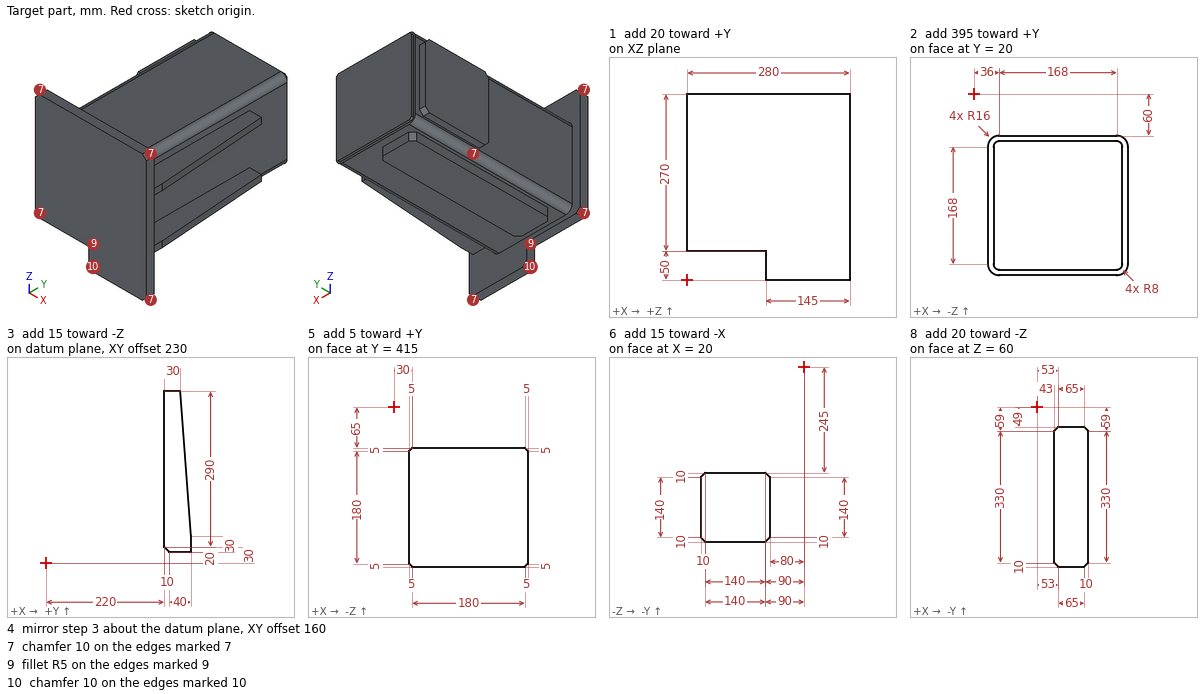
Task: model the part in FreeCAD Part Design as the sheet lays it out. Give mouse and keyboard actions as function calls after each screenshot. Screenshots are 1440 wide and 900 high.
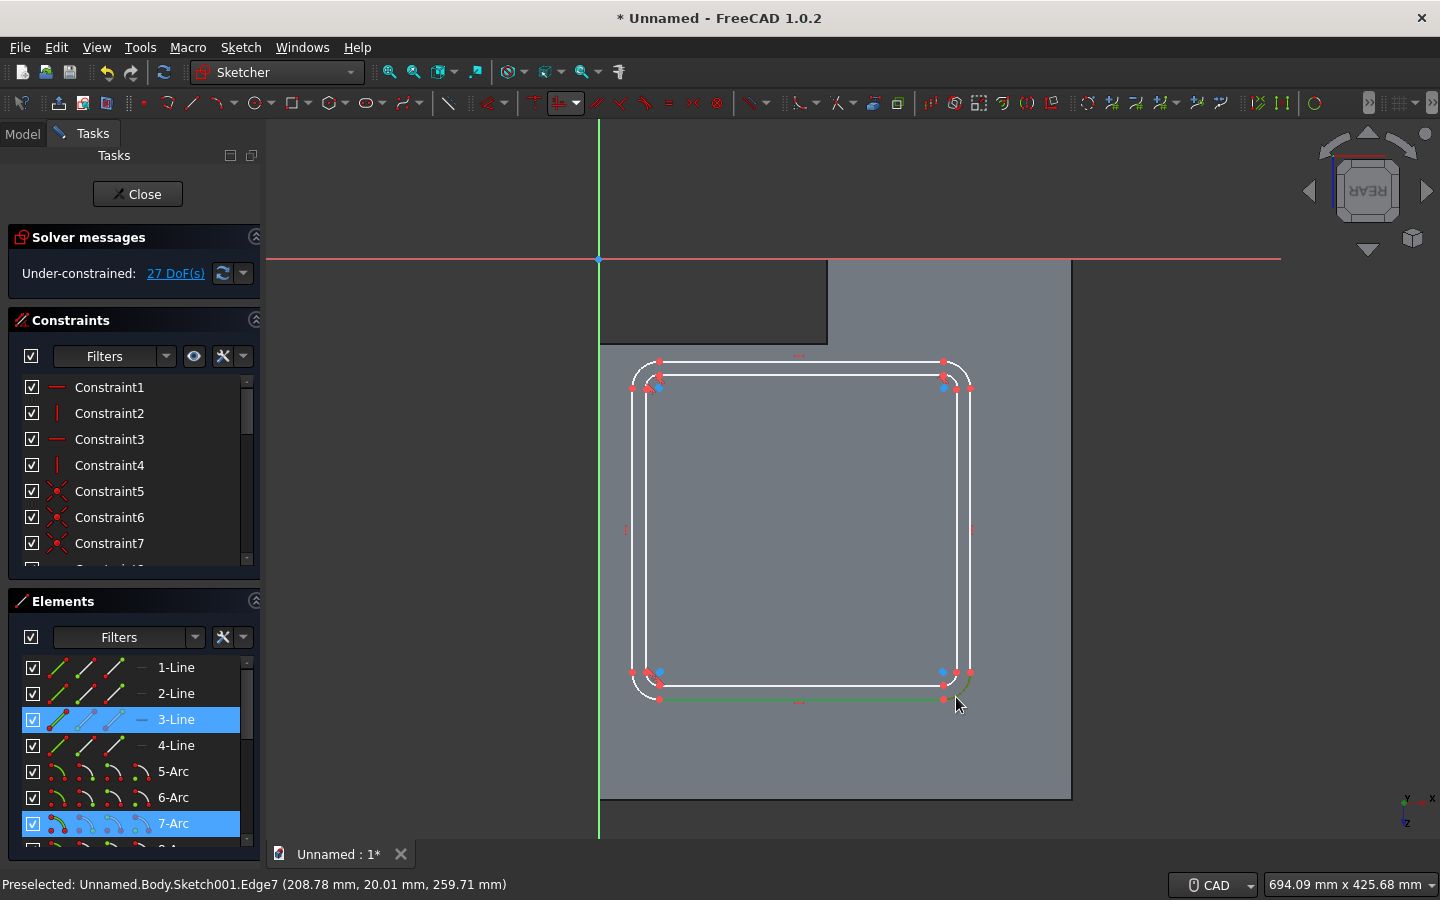
click(646, 104)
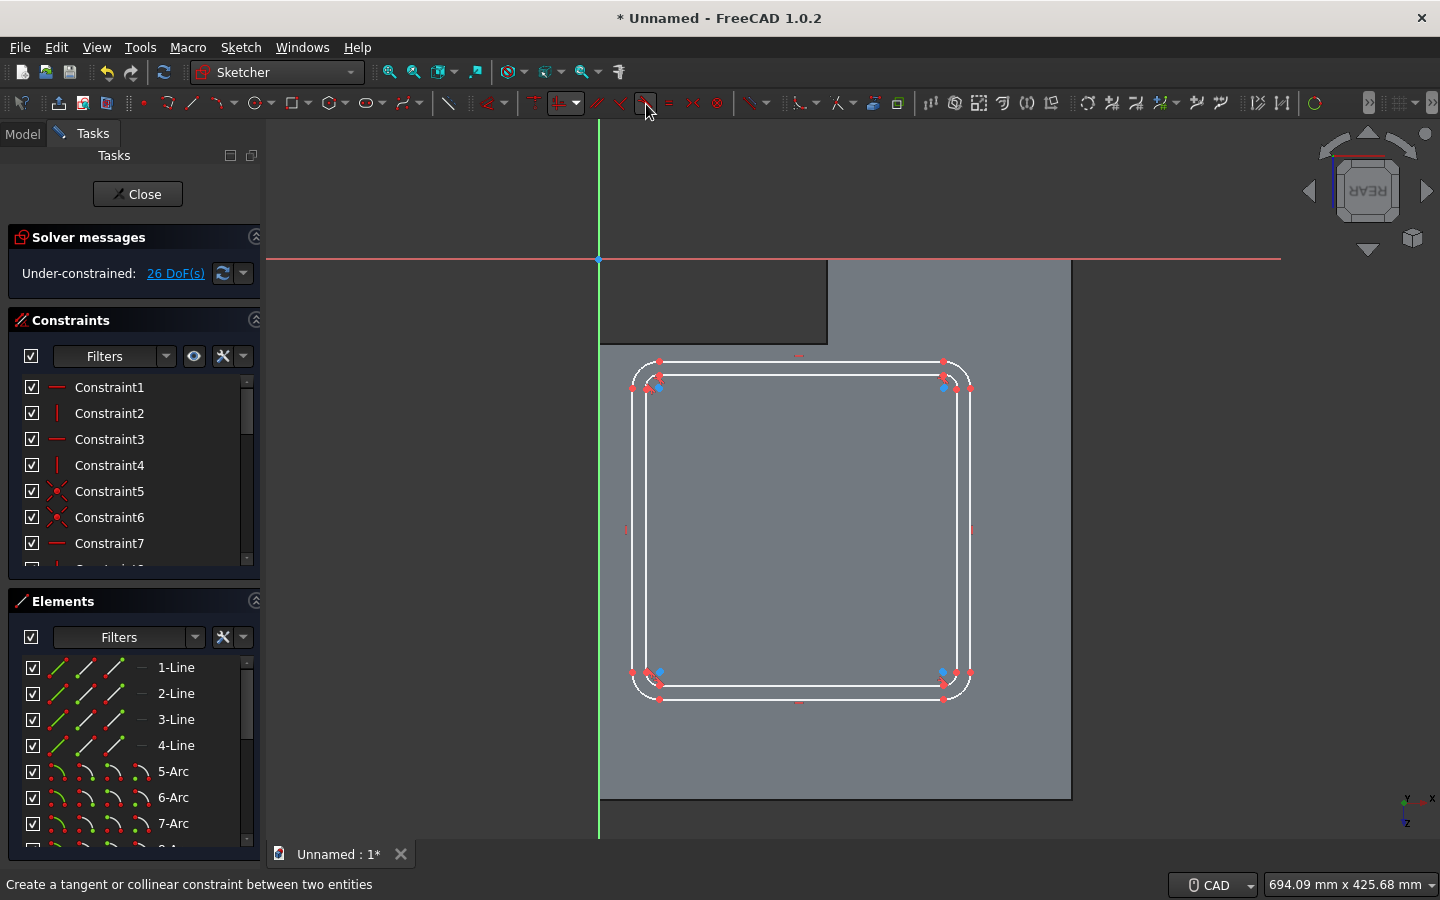
click(970, 588)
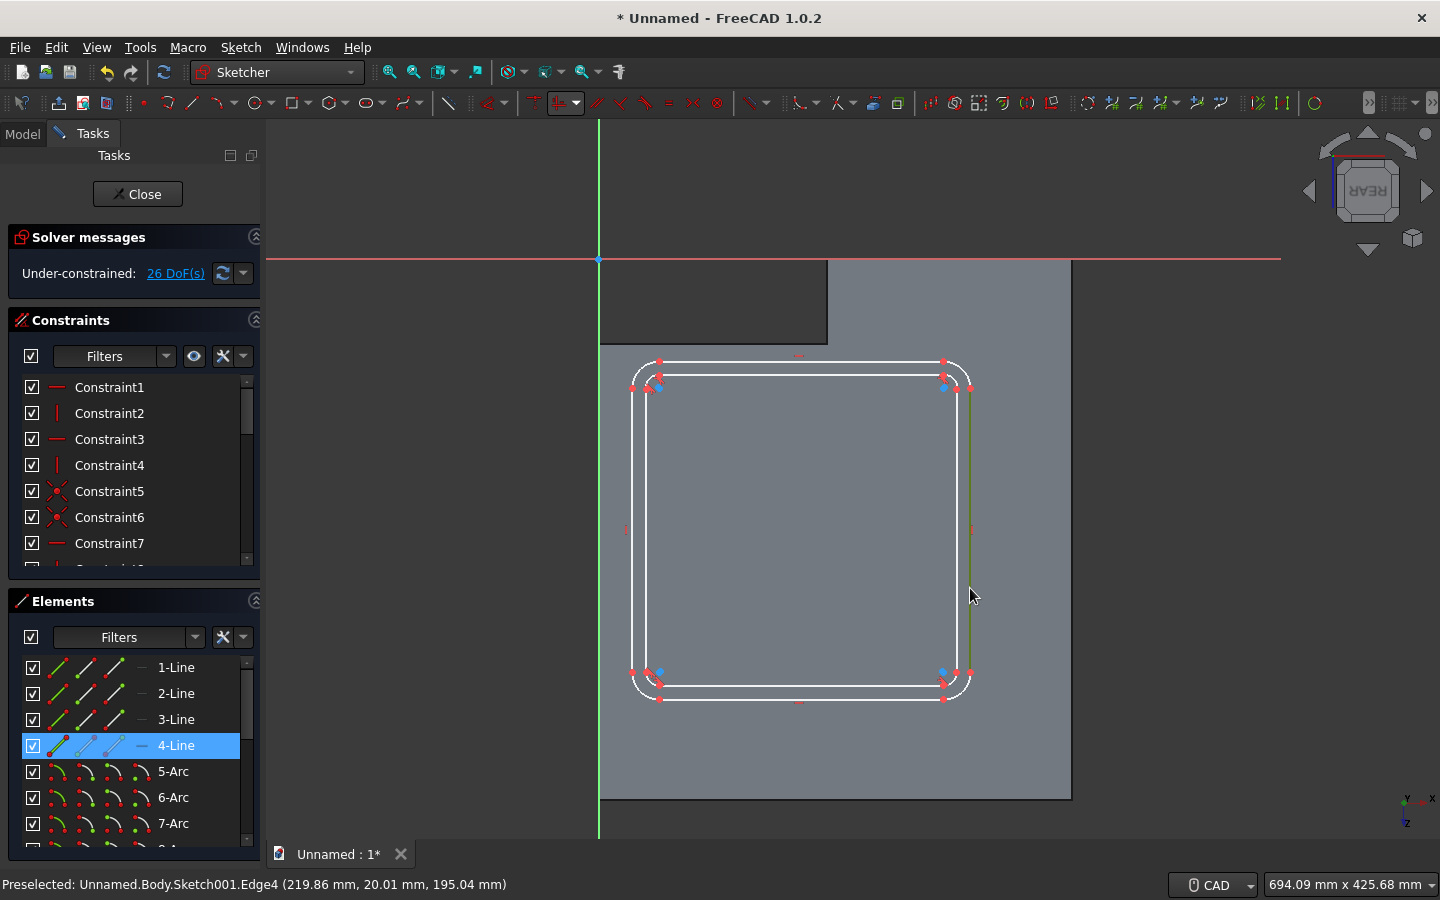
click(956, 697)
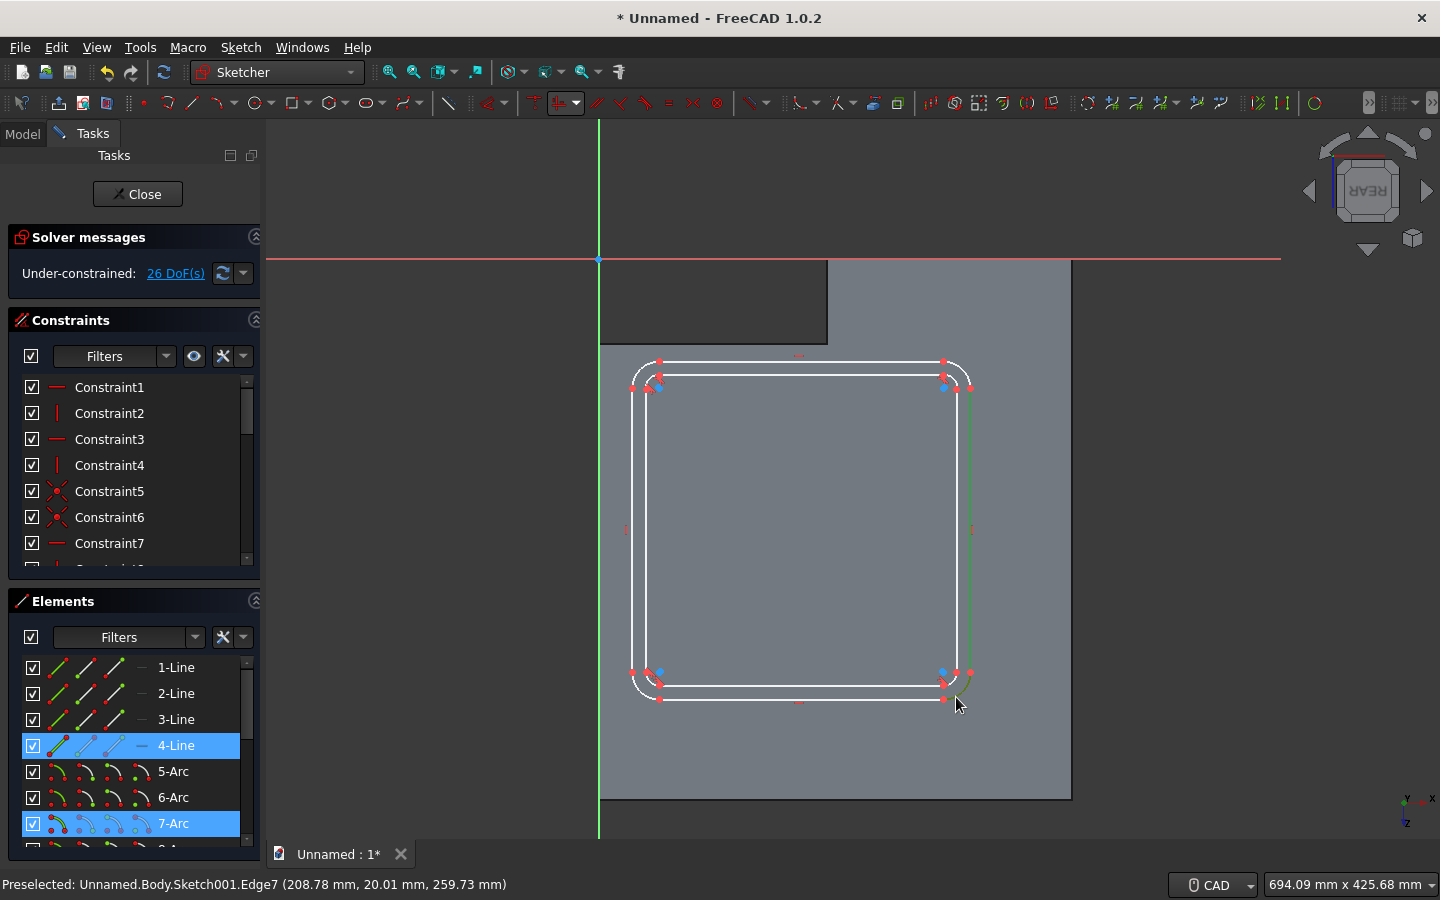
click(646, 104)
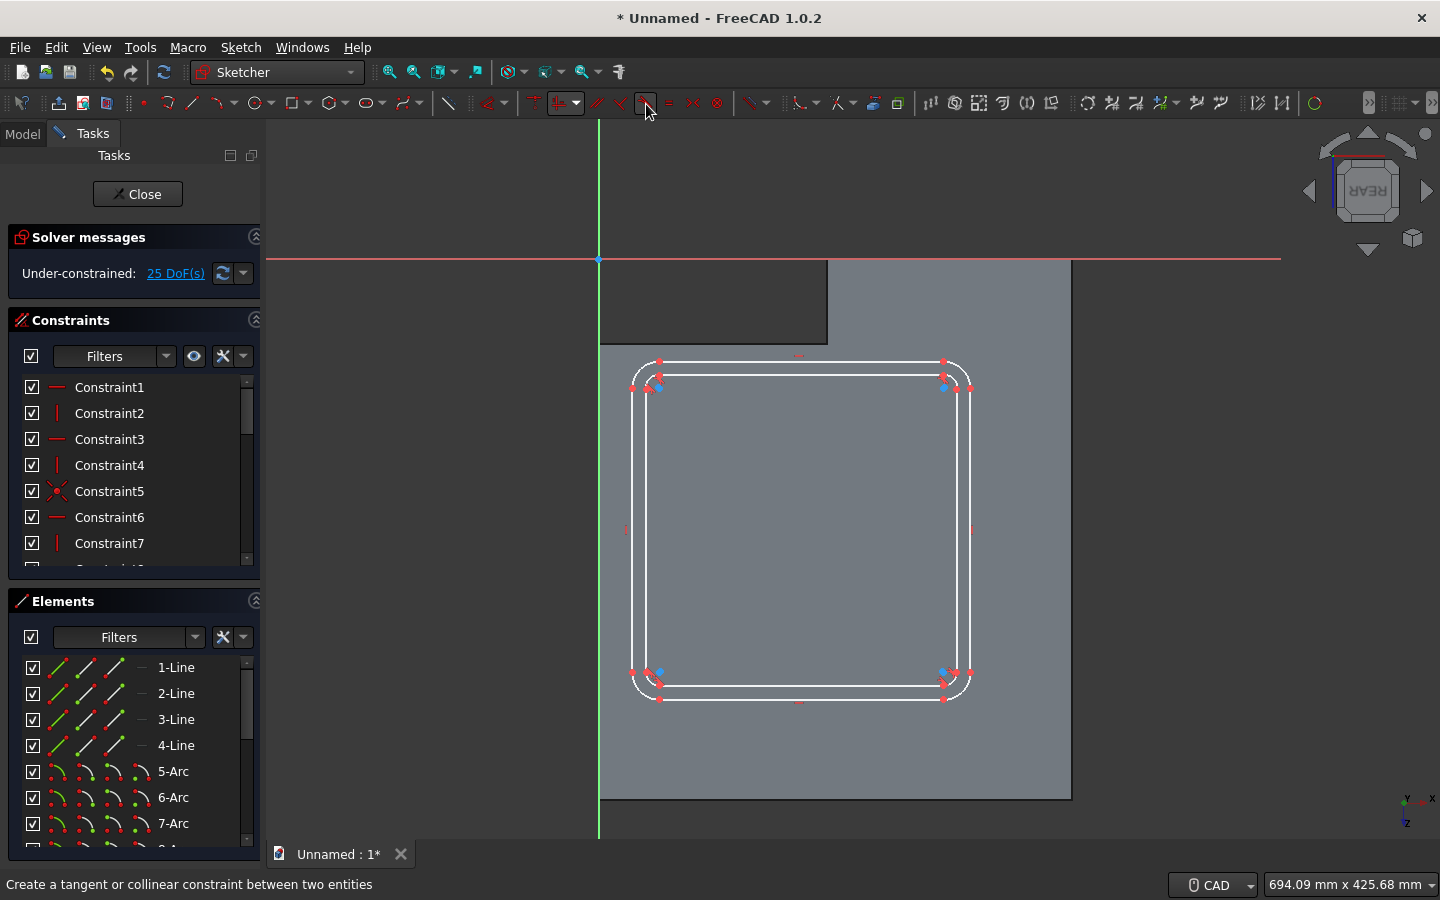
click(970, 588)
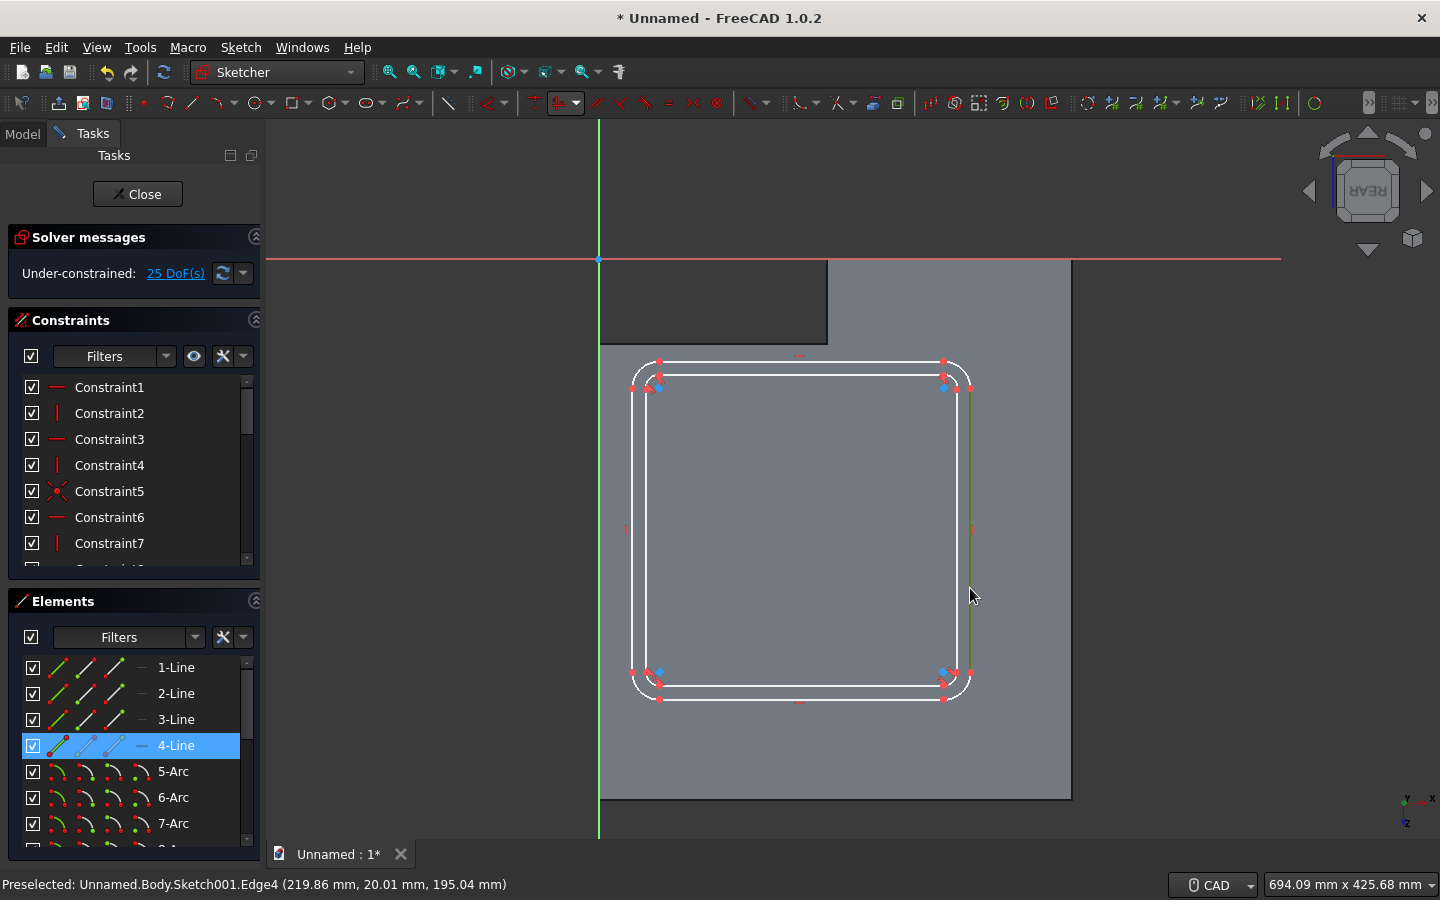
click(967, 376)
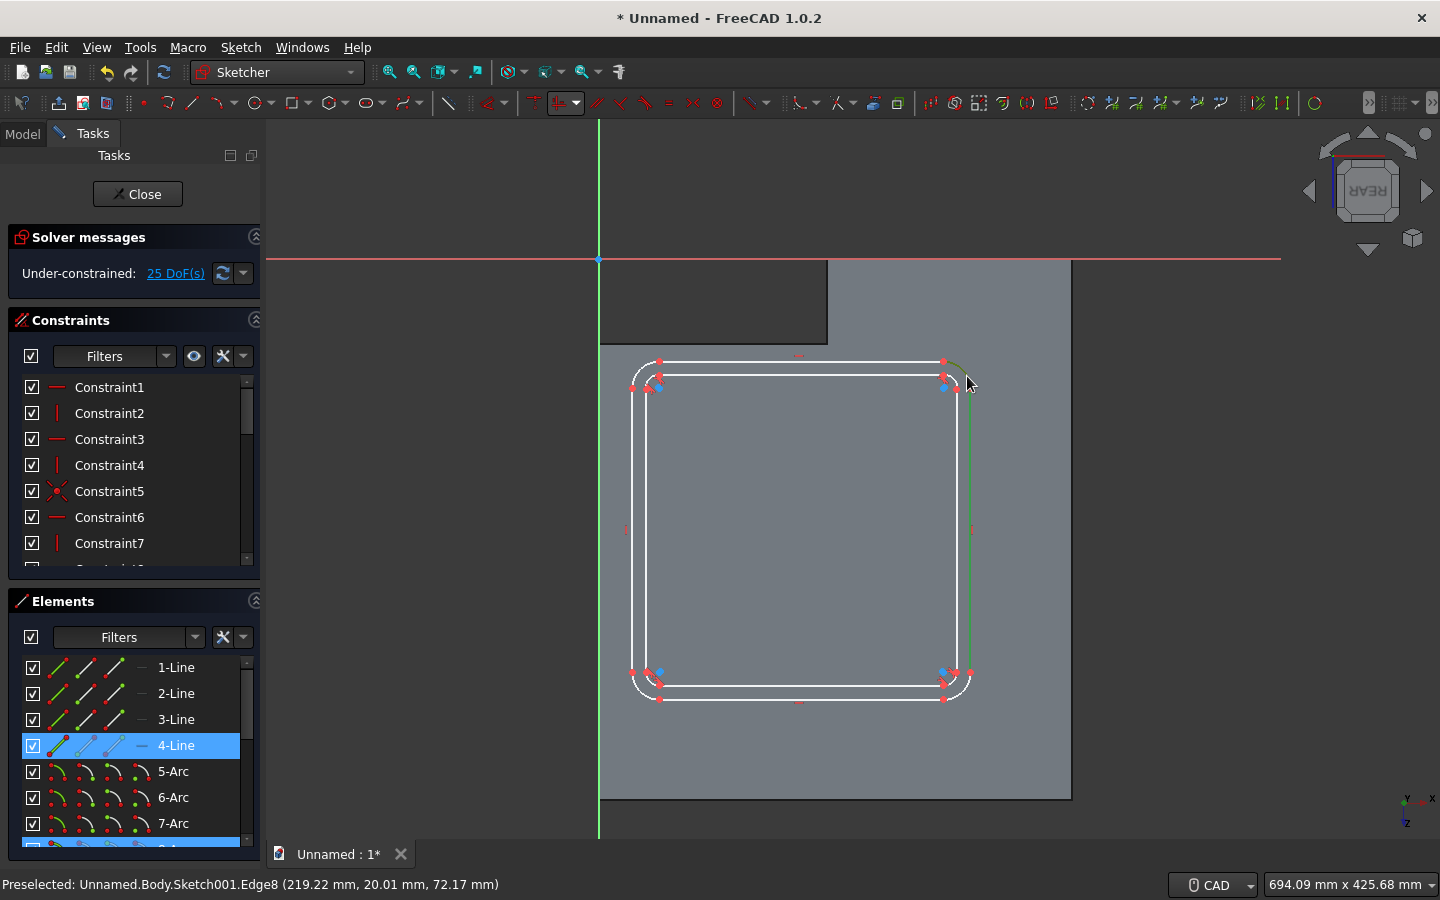
click(646, 104)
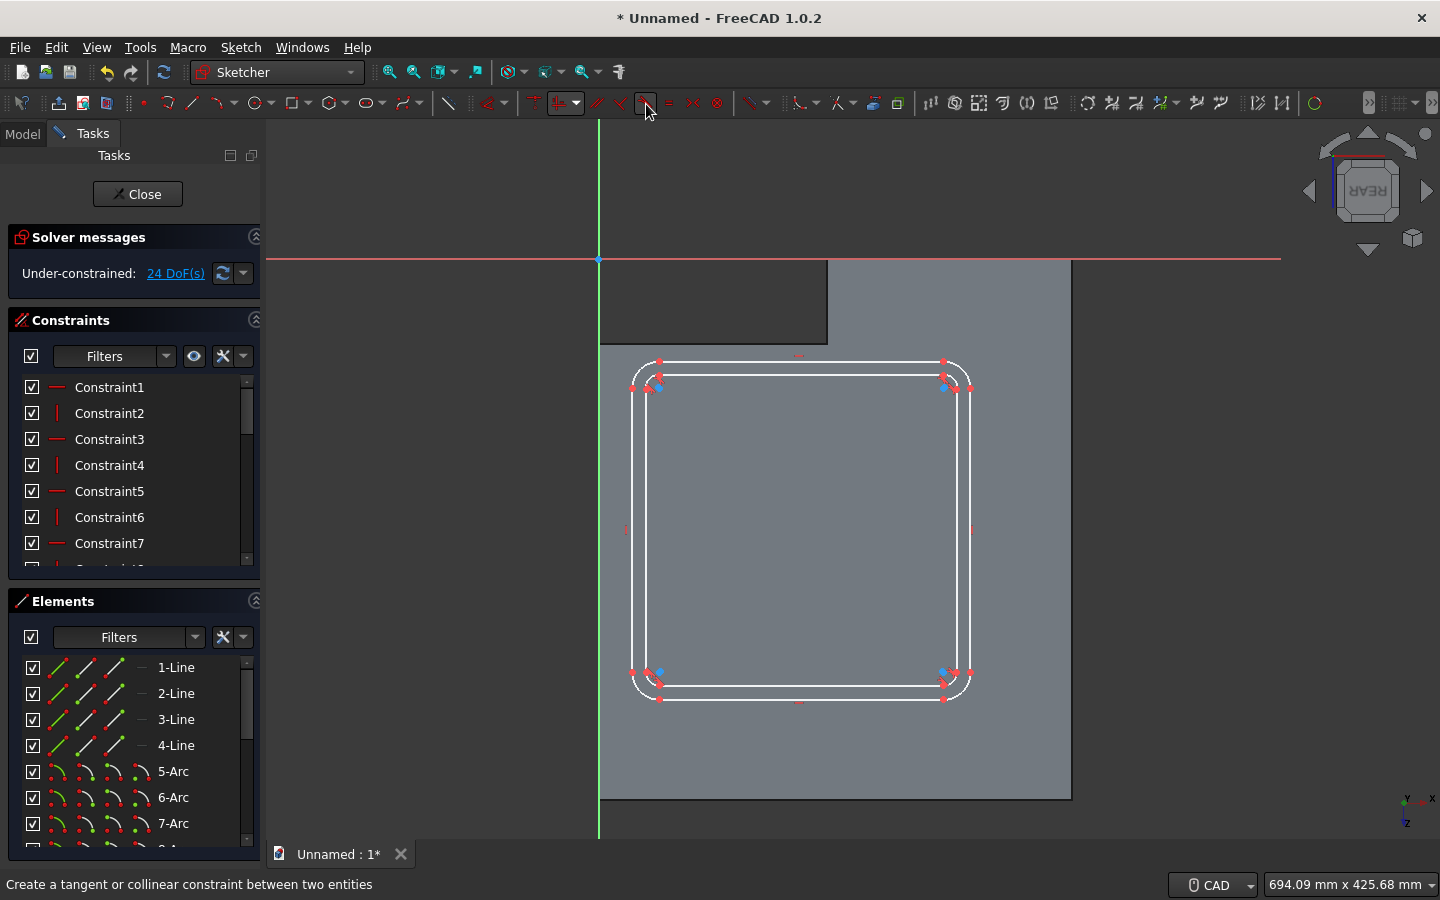
click(744, 375)